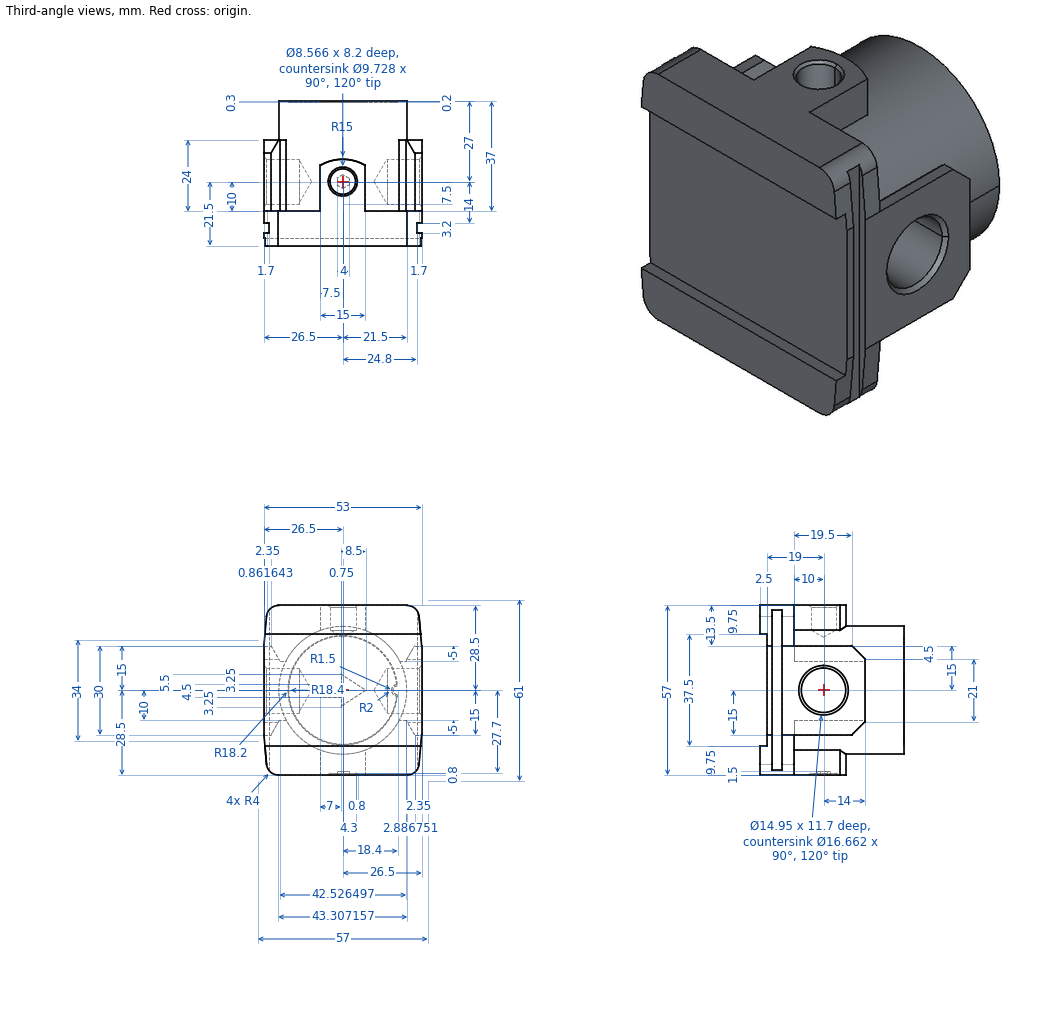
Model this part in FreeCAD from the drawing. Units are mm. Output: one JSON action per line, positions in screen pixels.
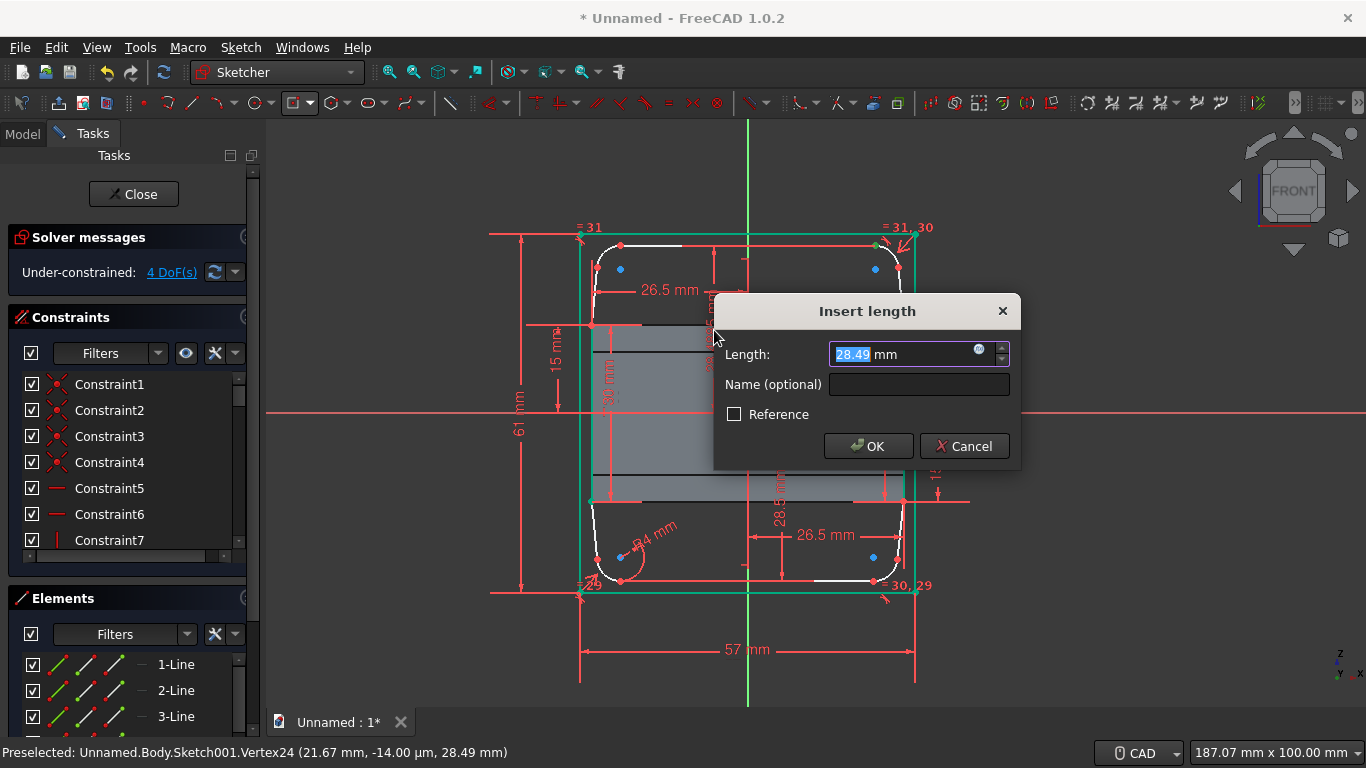
{"action": "type", "text": "28.5"}
{"action": "key", "text": "Return"}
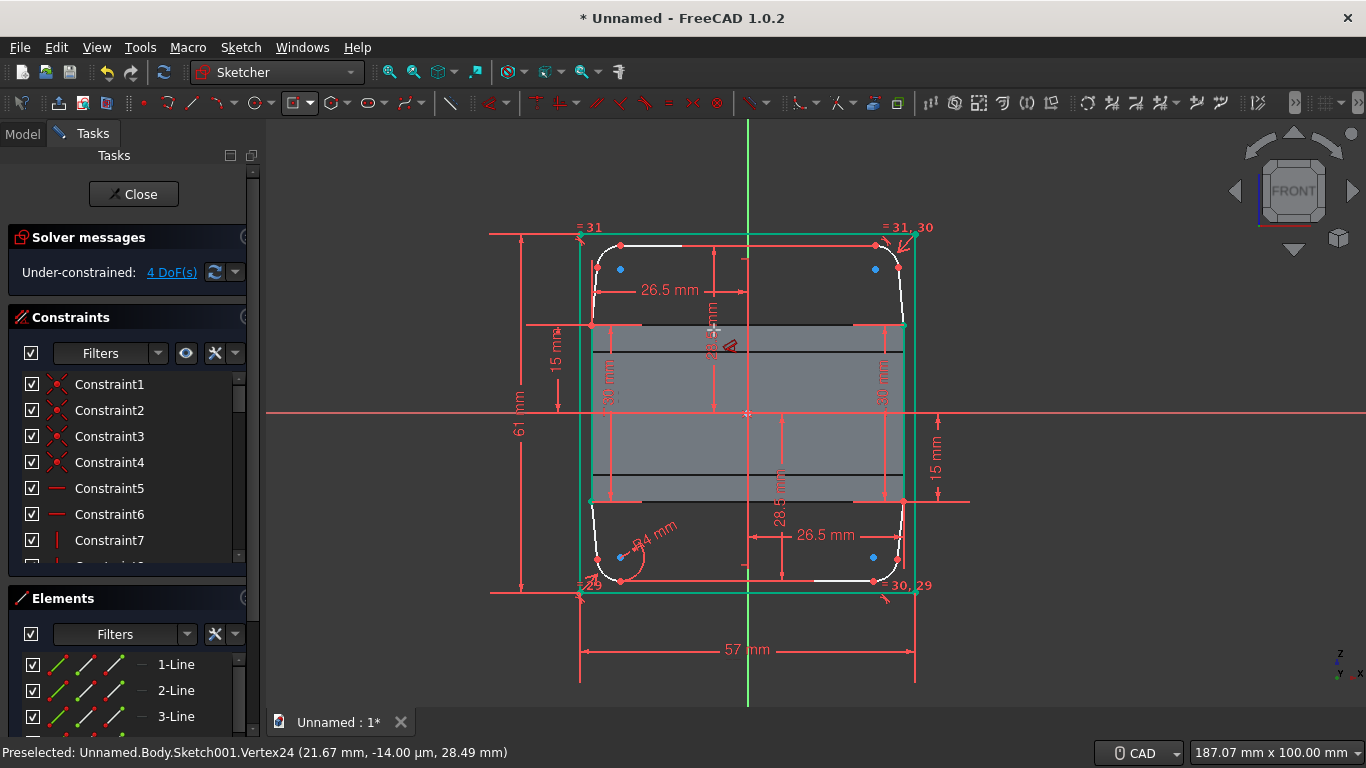
{"action": "left_click", "coordinate": [697, 581]}
{"action": "left_click", "coordinate": [689, 615]}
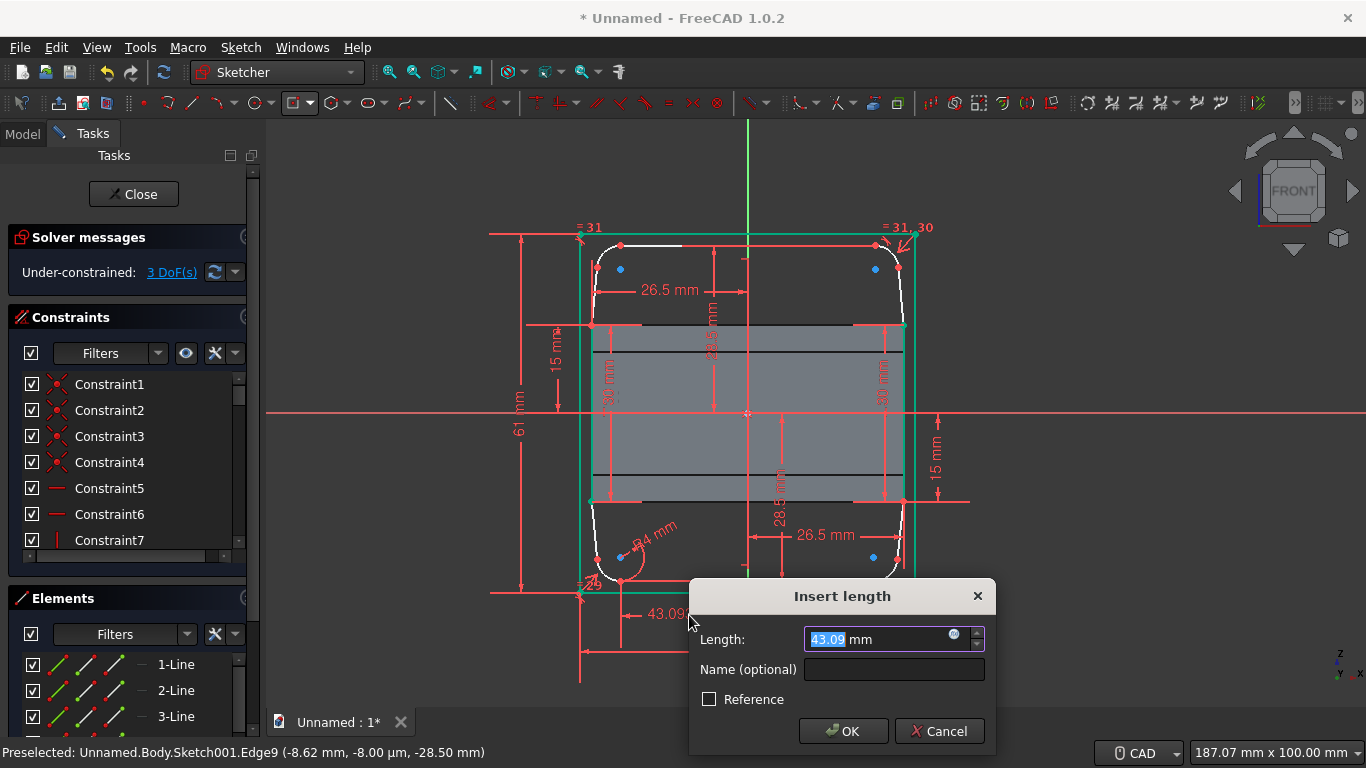
{"action": "type", "text": "43.307157"}
{"action": "key", "text": "Return"}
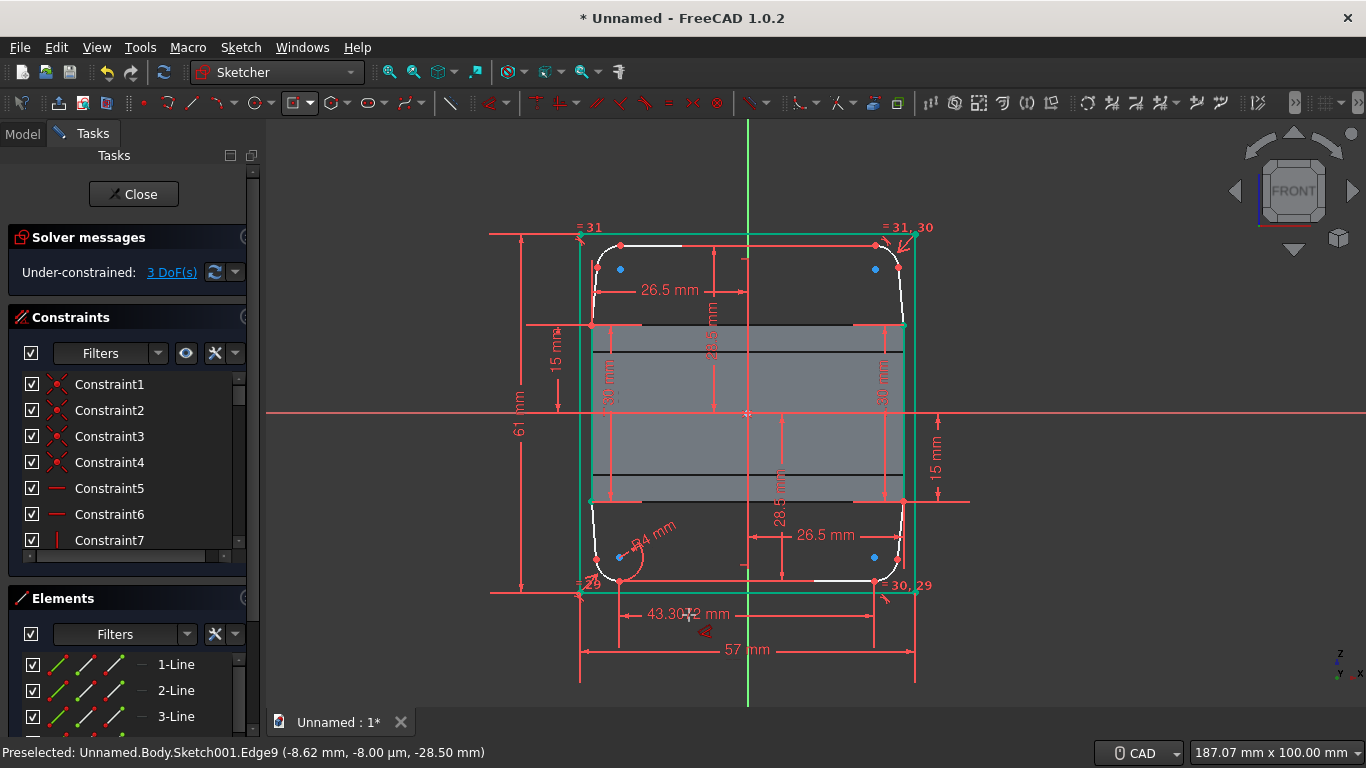
{"action": "left_click", "coordinate": [799, 246]}
{"action": "left_click", "coordinate": [689, 212]}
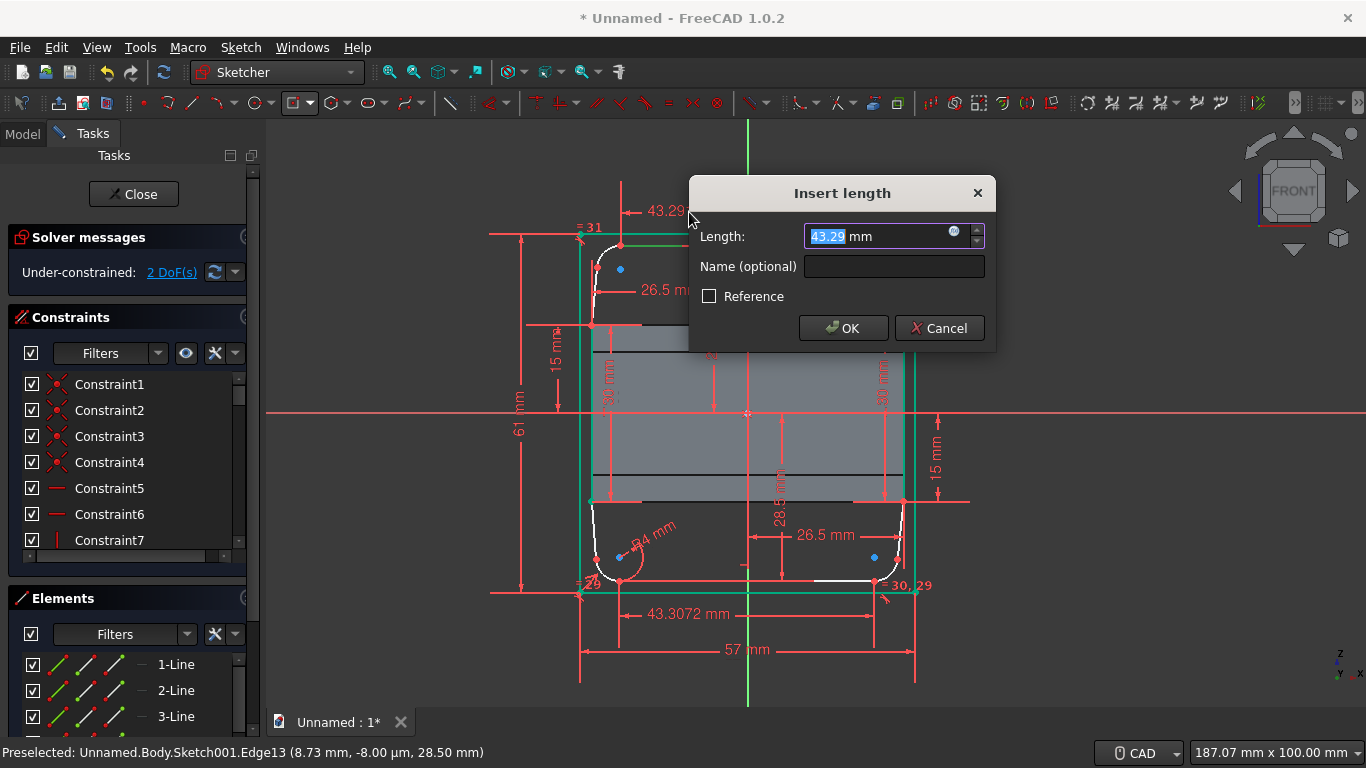
{"action": "type", "text": "43.307157"}
{"action": "key", "text": "Return"}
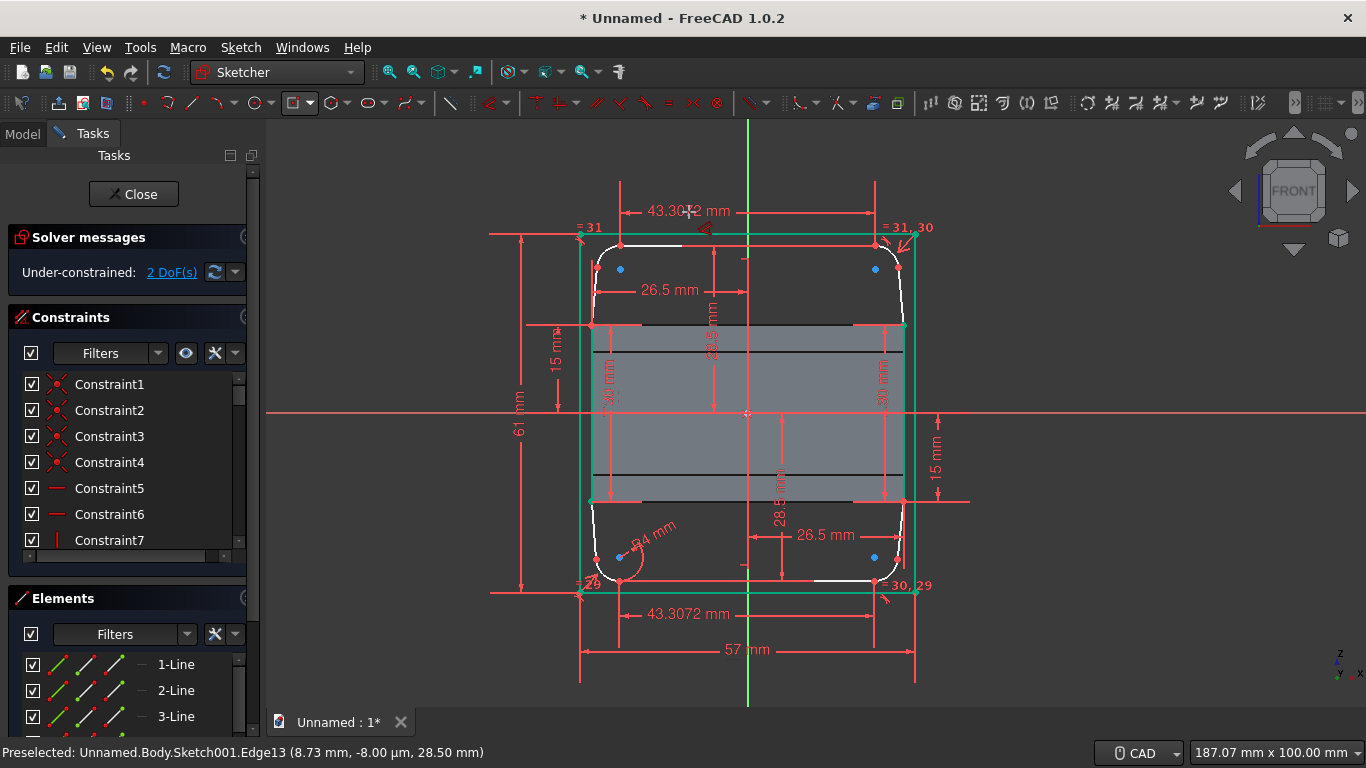
{"action": "scroll", "coordinate": [595, 285], "scroll_direction": "up", "scroll_amount": 11}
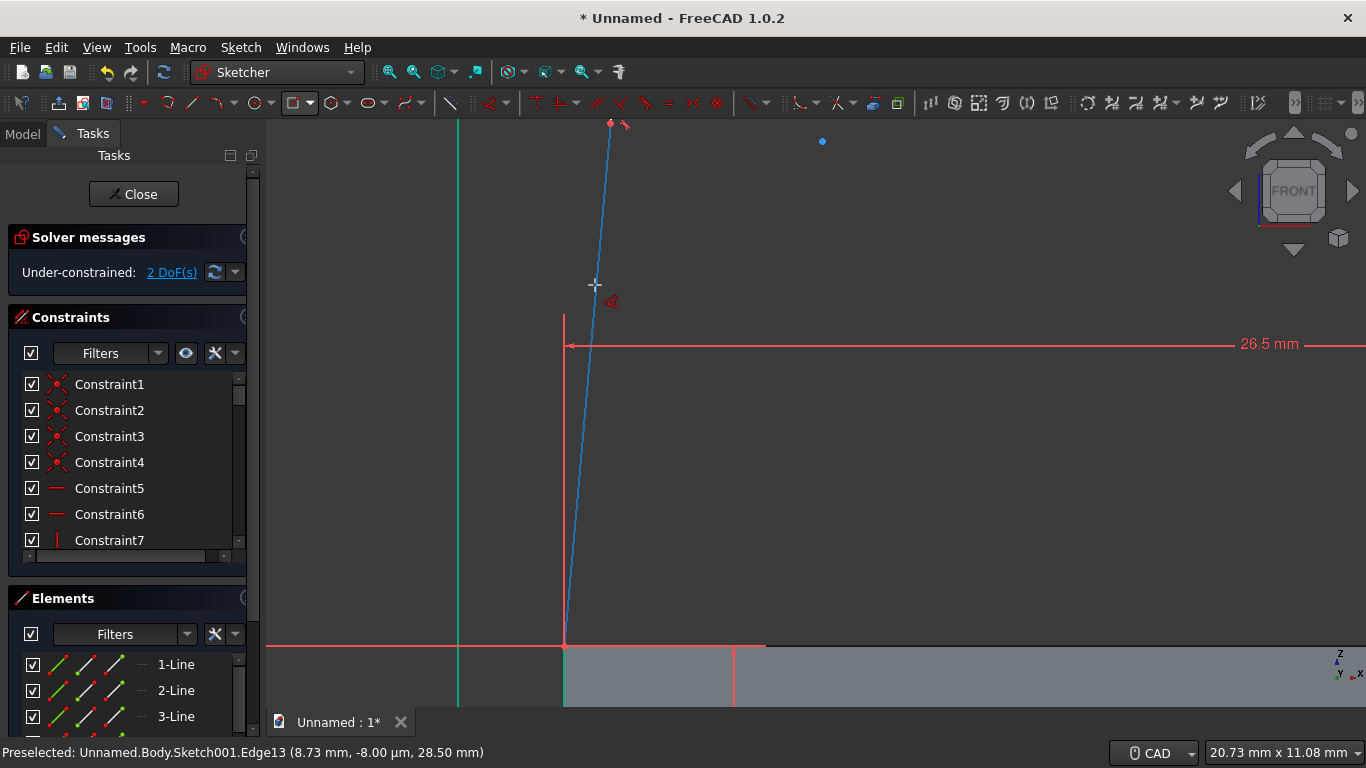
{"action": "left_click", "coordinate": [597, 280]}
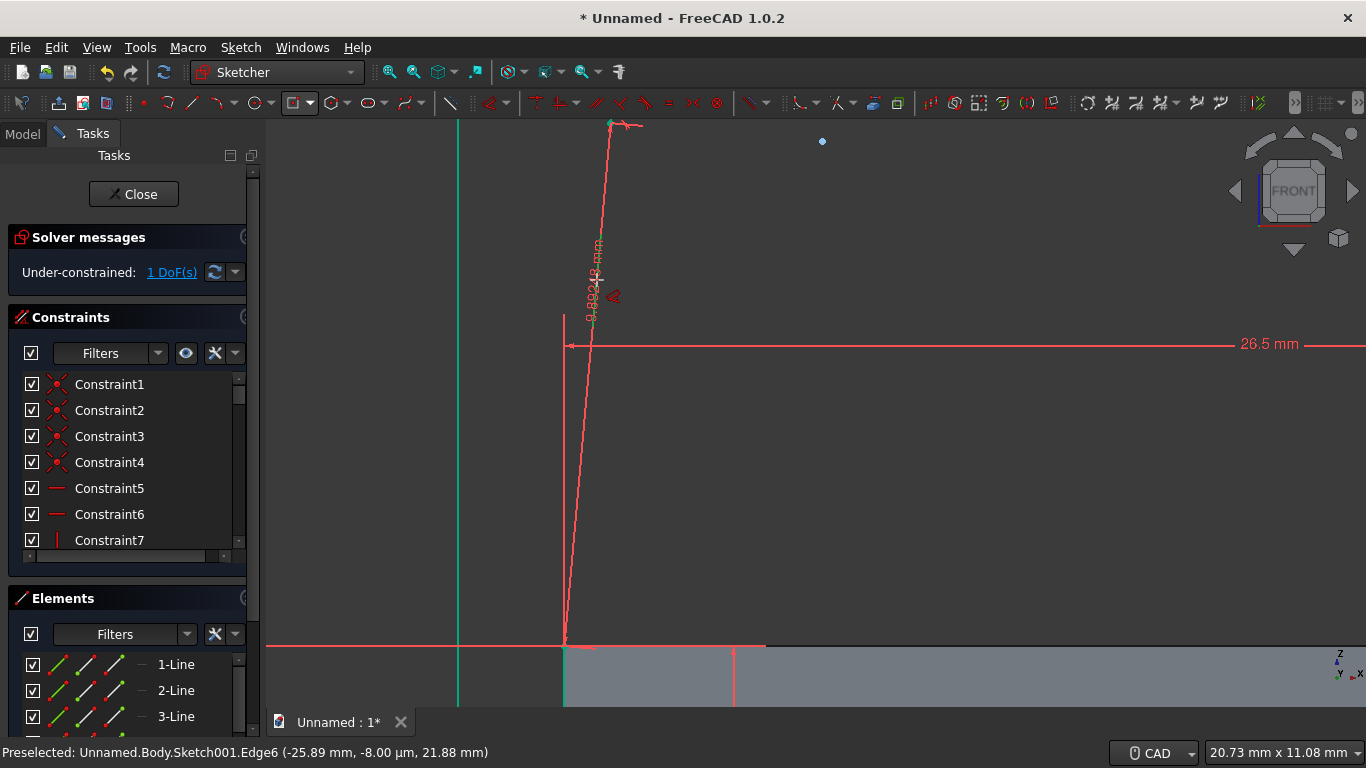
{"action": "key", "text": "Escape"}
{"action": "key", "text": "Escape"}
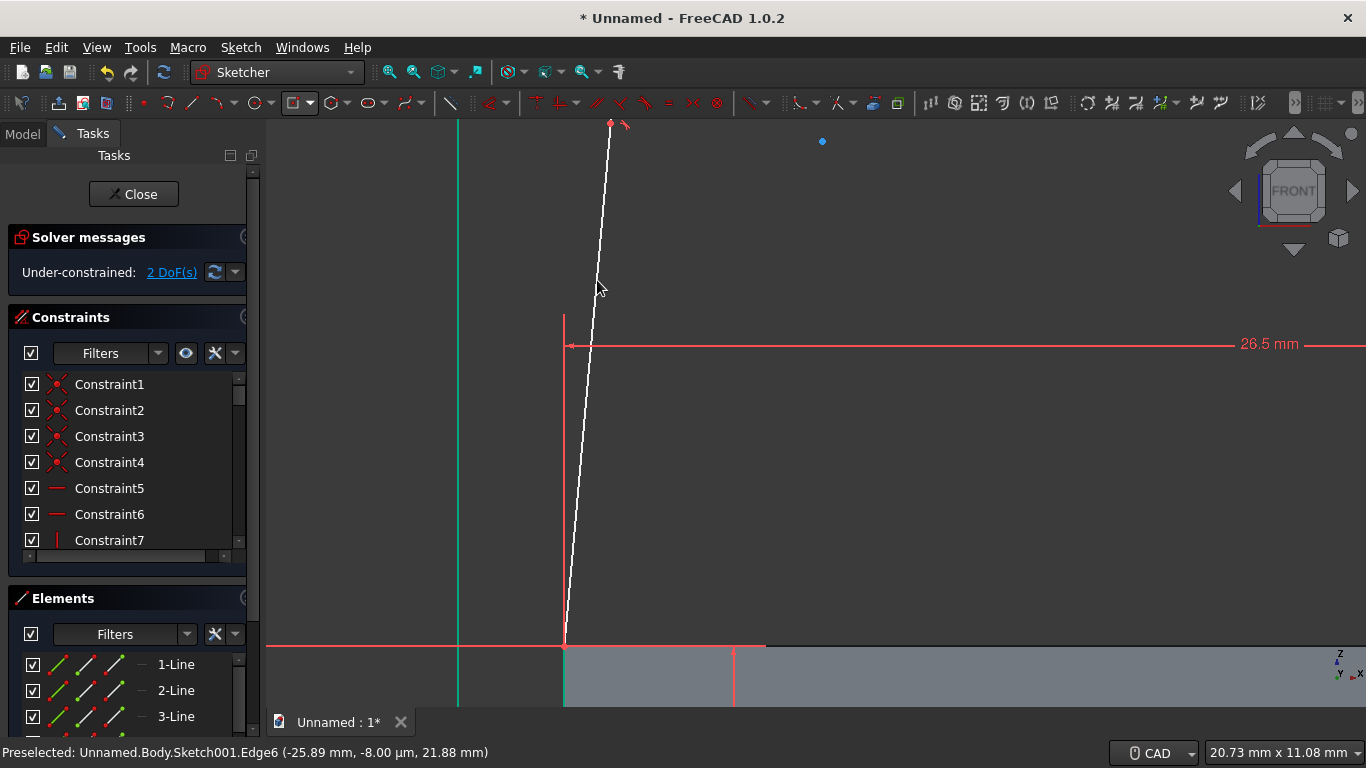
{"action": "left_click", "coordinate": [597, 280]}